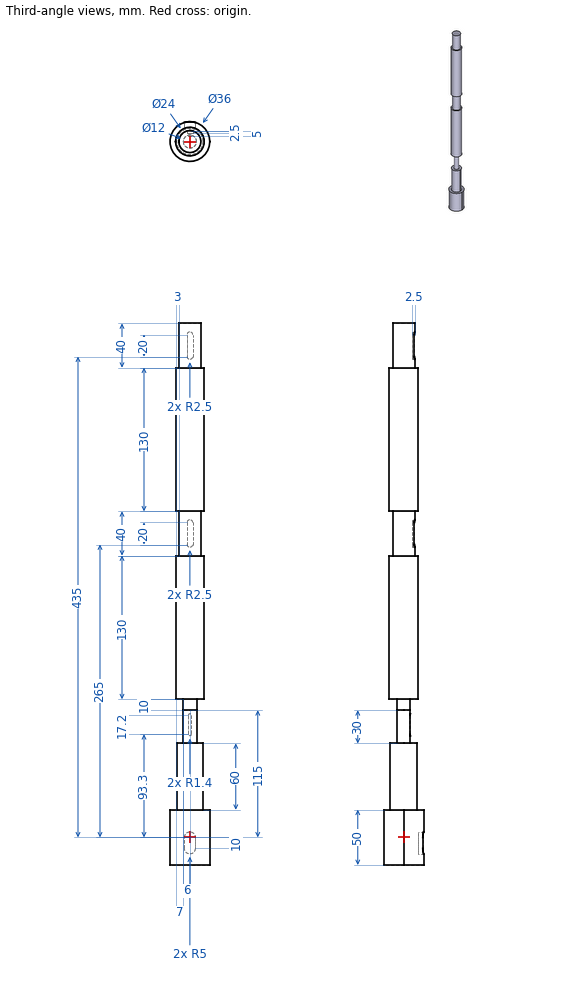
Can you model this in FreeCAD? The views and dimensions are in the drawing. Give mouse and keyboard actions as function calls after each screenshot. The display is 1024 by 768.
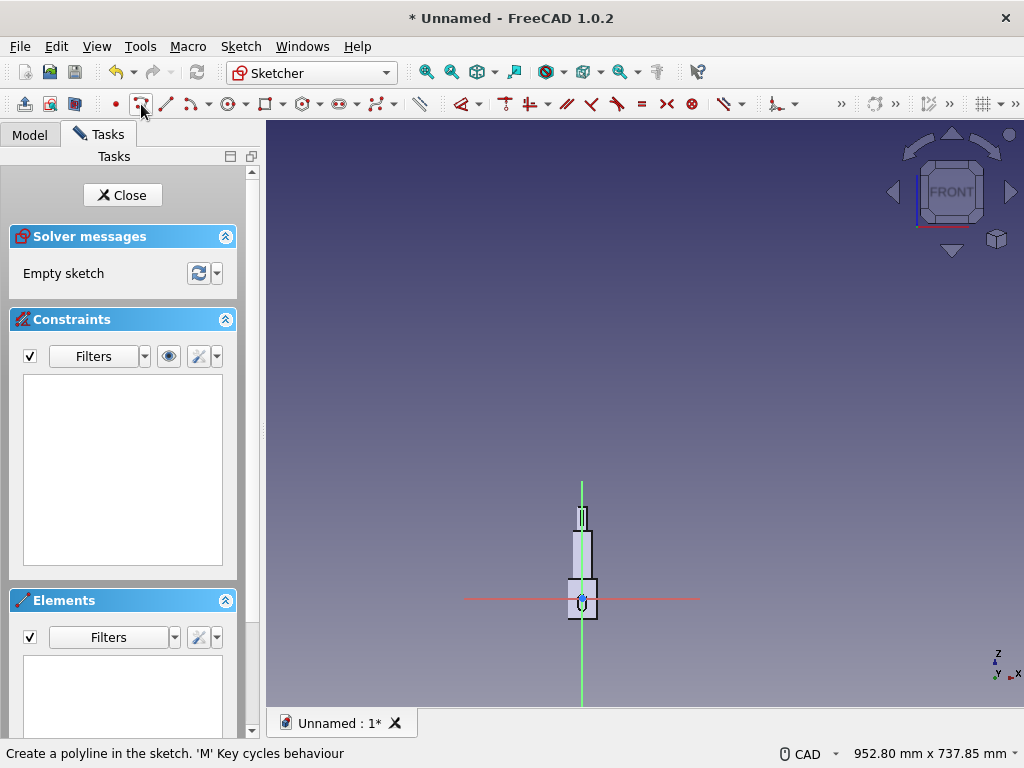
click(582, 507)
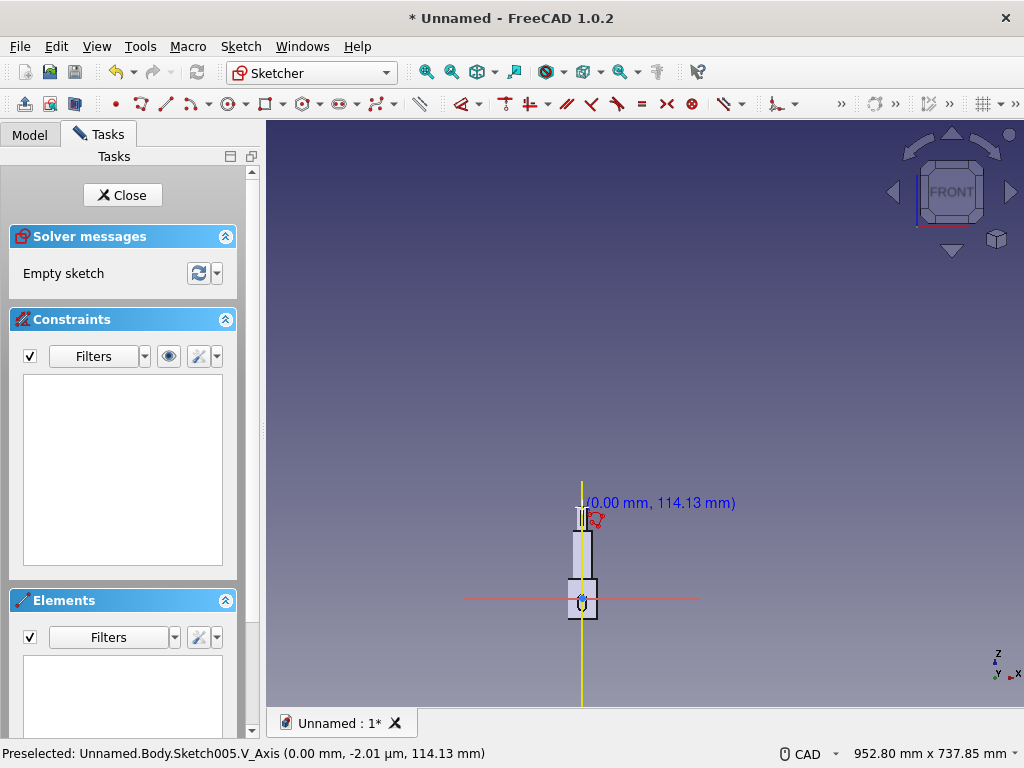
scroll(577, 507, up, 7)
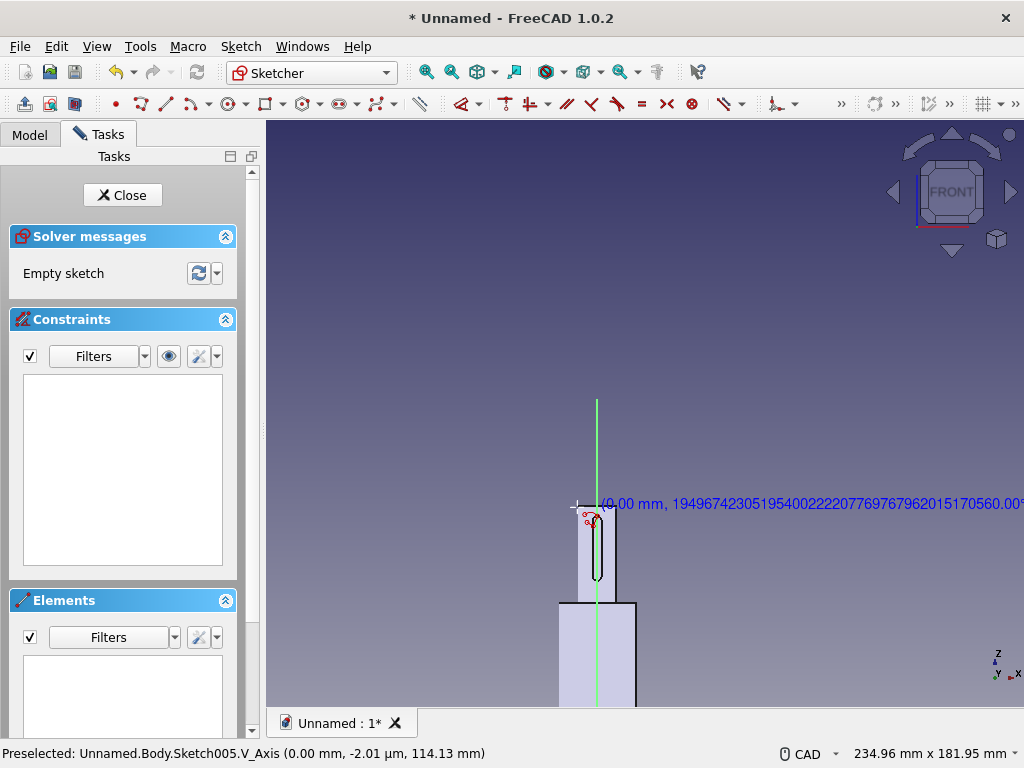
click(578, 505)
click(578, 474)
click(555, 474)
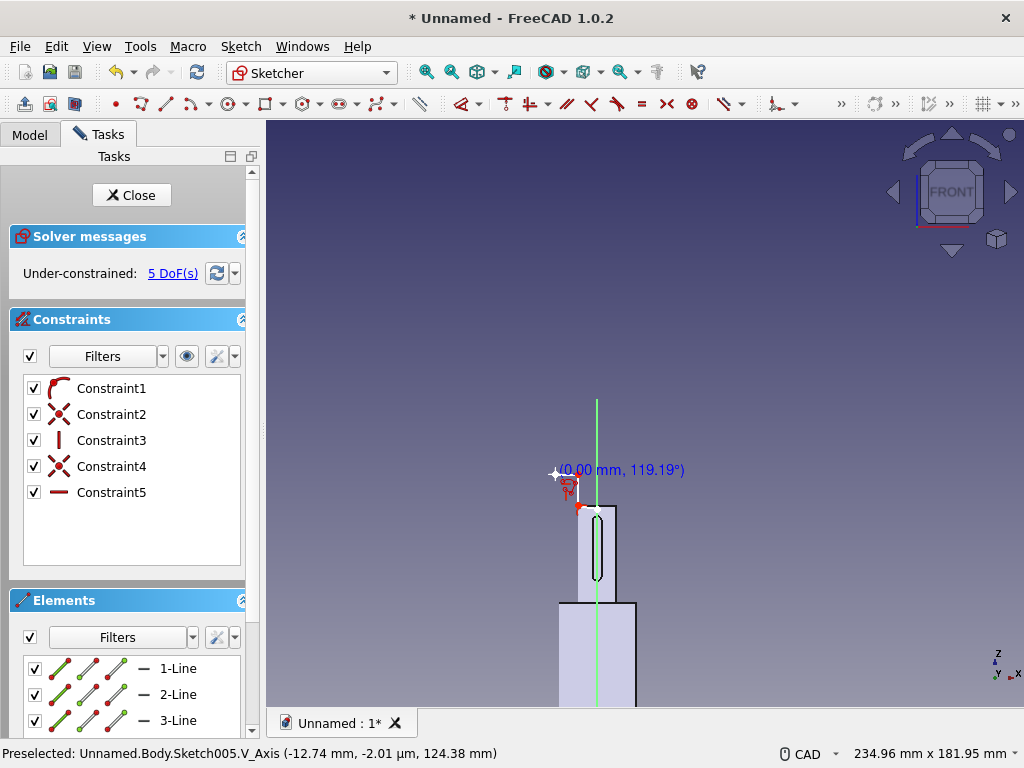
scroll(577, 507, down, 7)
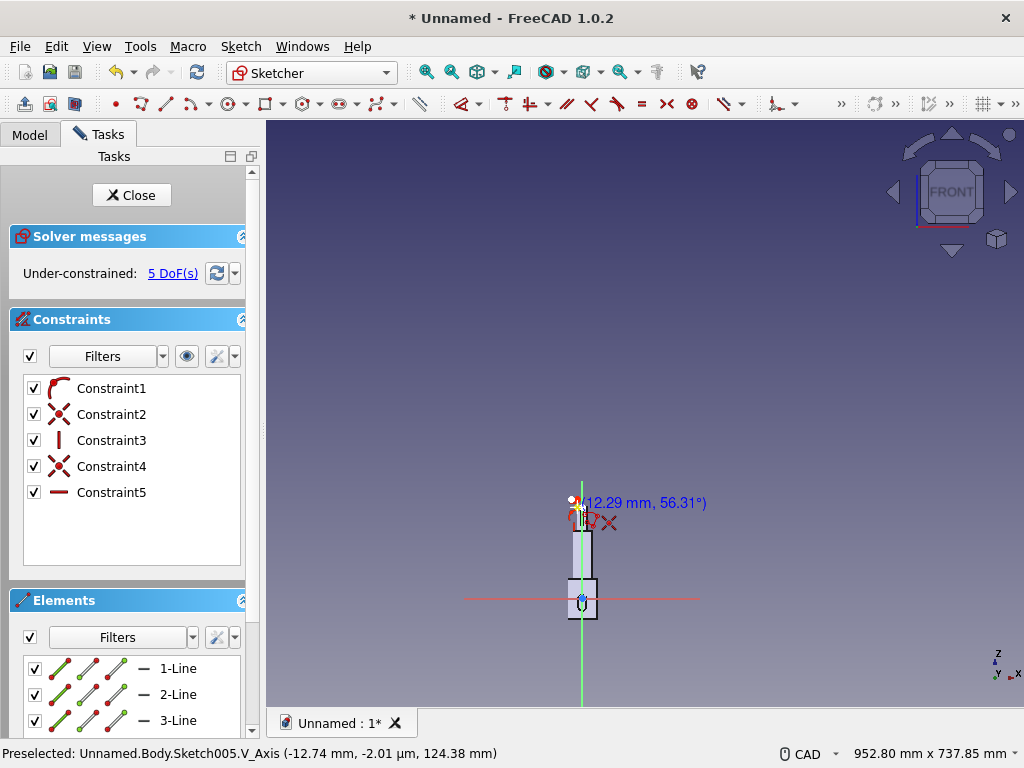
scroll(572, 396, up, 3)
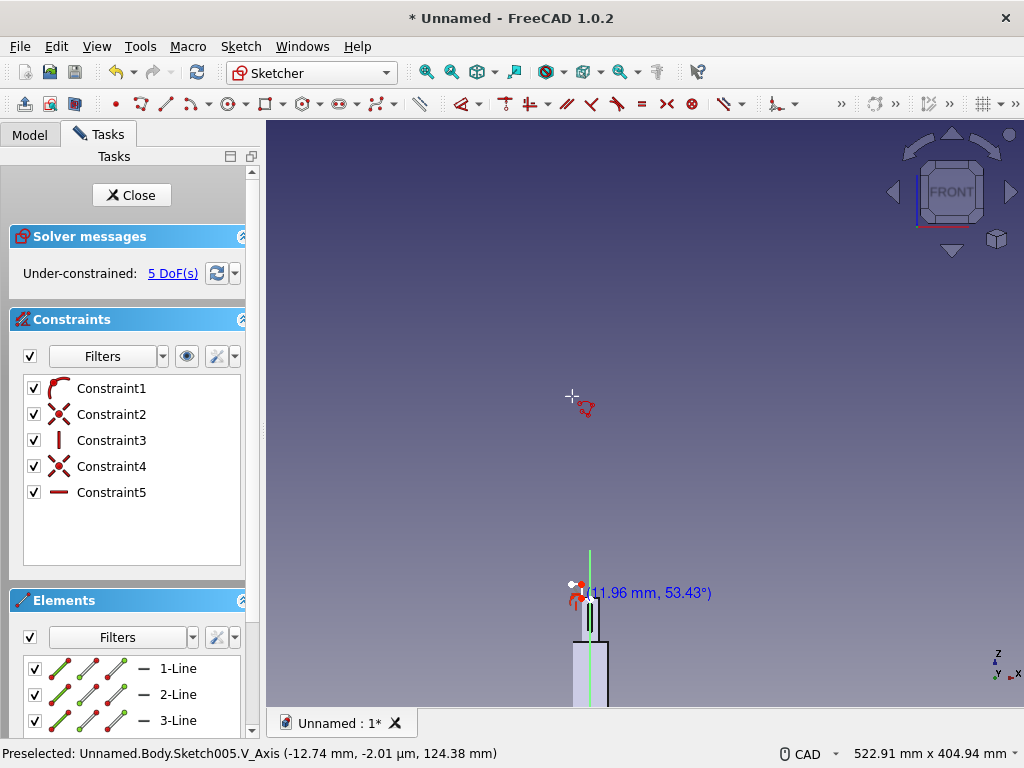
click(571, 395)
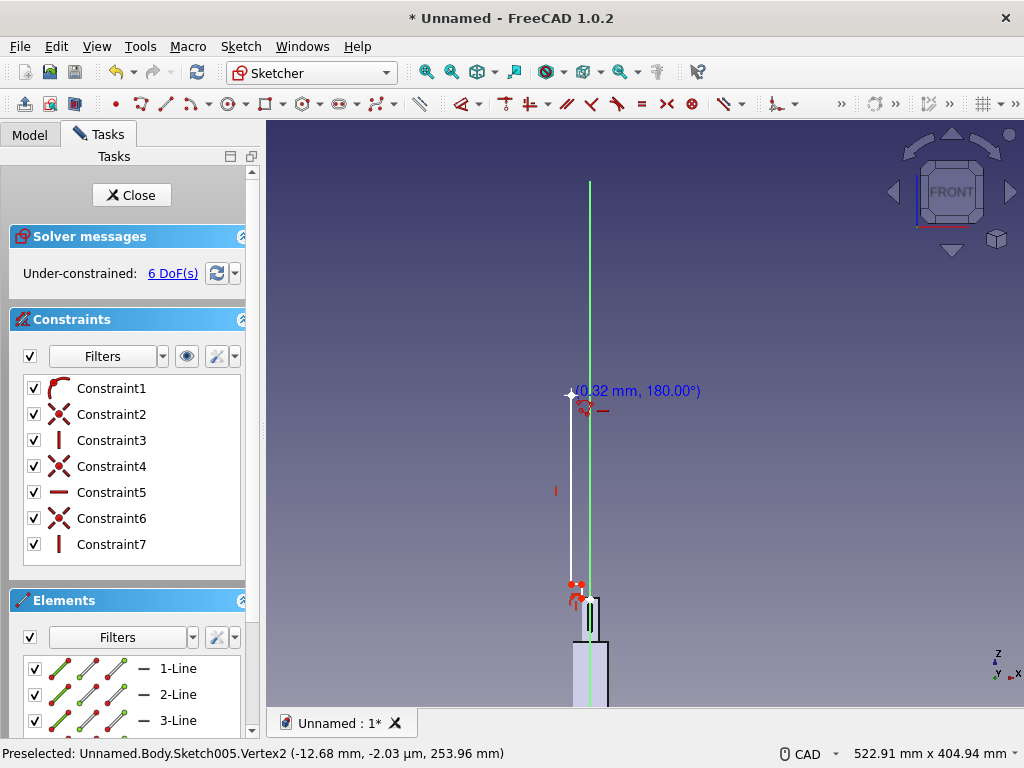
scroll(576, 395, up, 7)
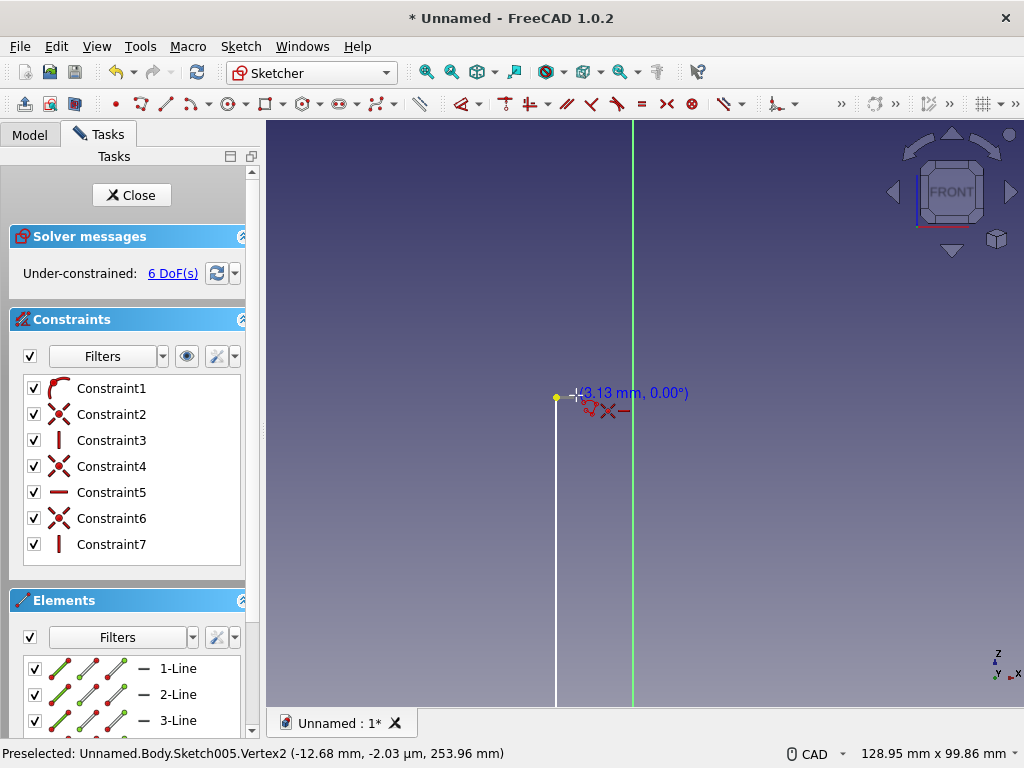
click(574, 394)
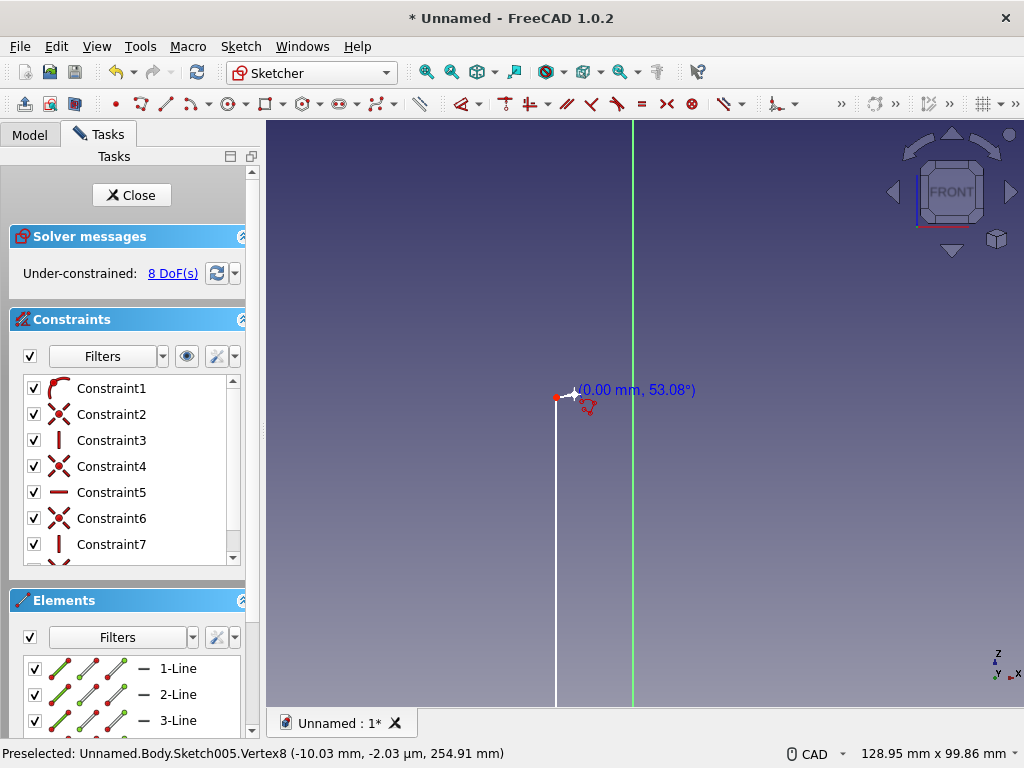
scroll(574, 396, down, 10)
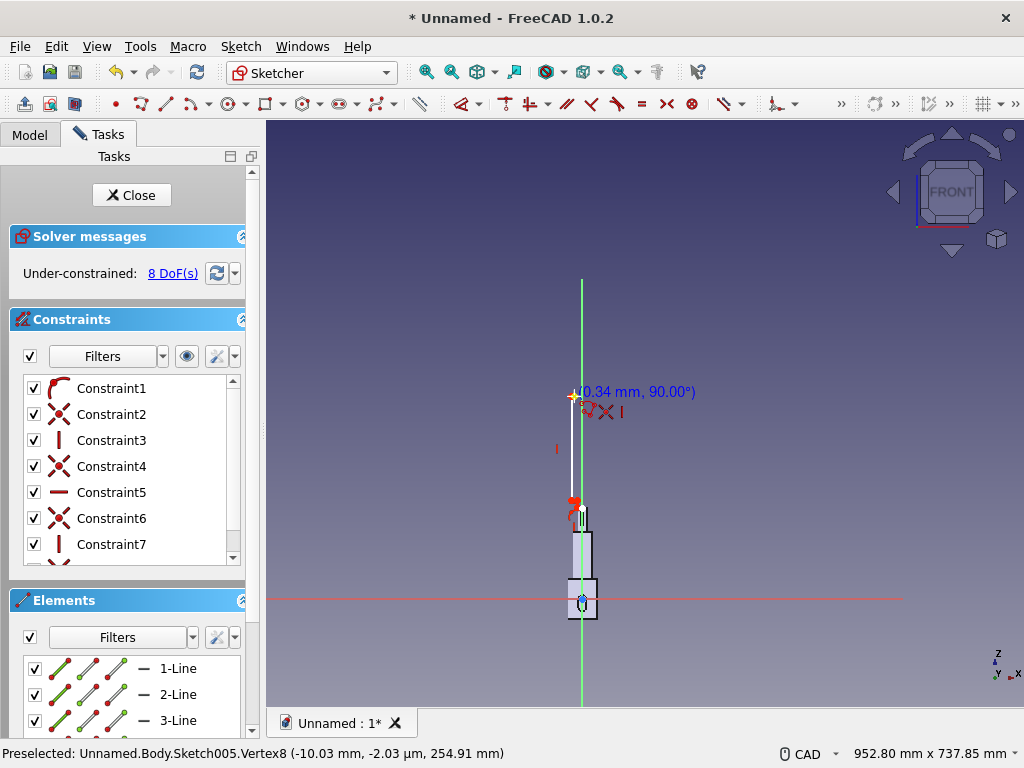
scroll(574, 365, up, 4)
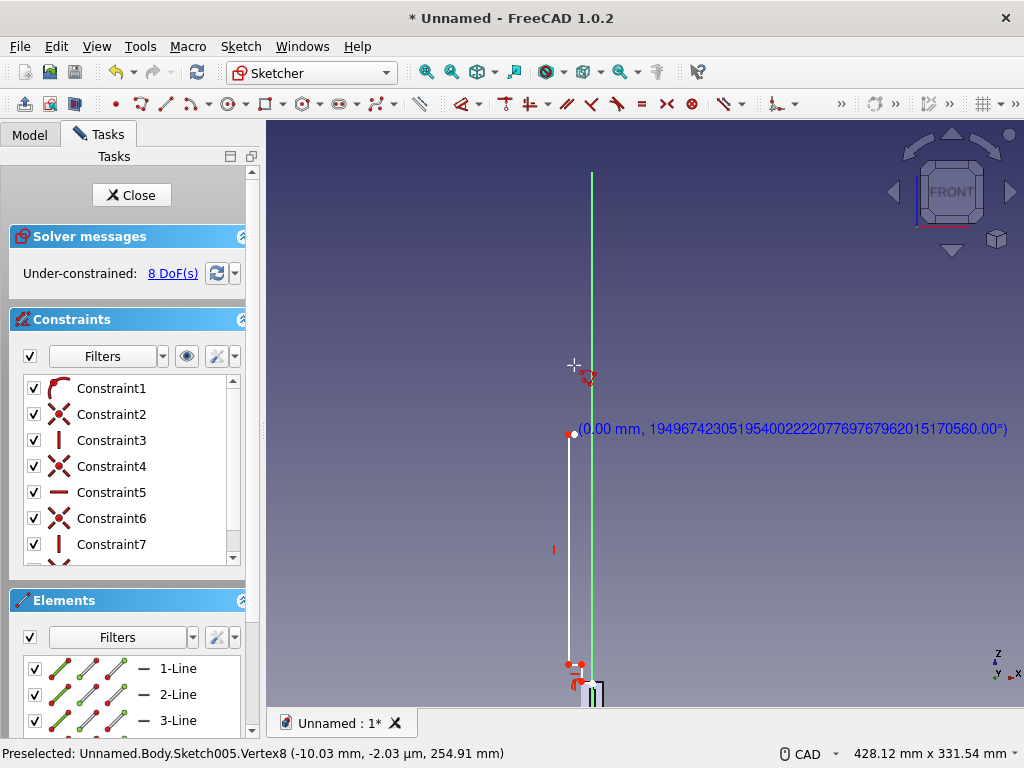
click(574, 363)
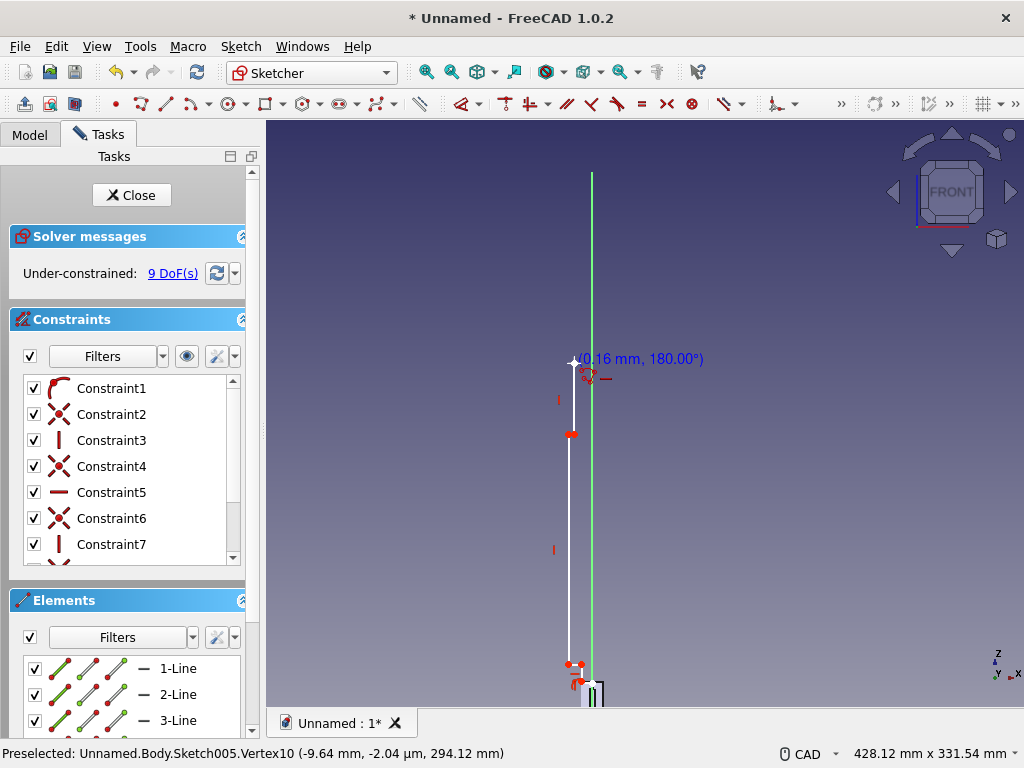
scroll(569, 363, up, 6)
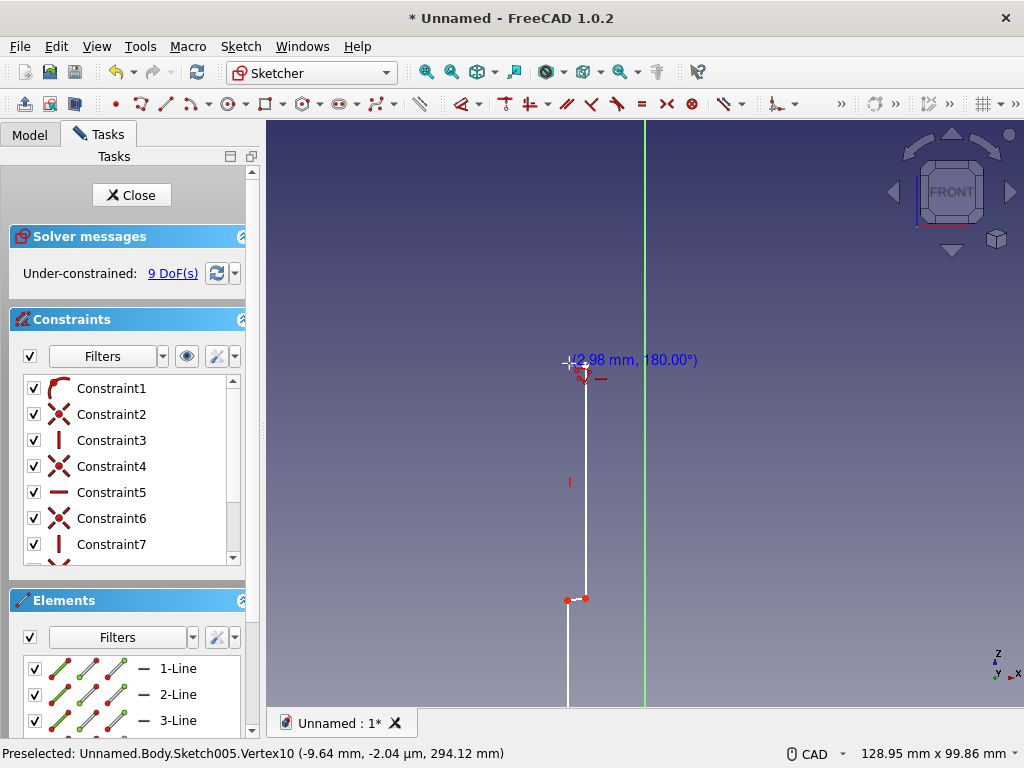
click(568, 362)